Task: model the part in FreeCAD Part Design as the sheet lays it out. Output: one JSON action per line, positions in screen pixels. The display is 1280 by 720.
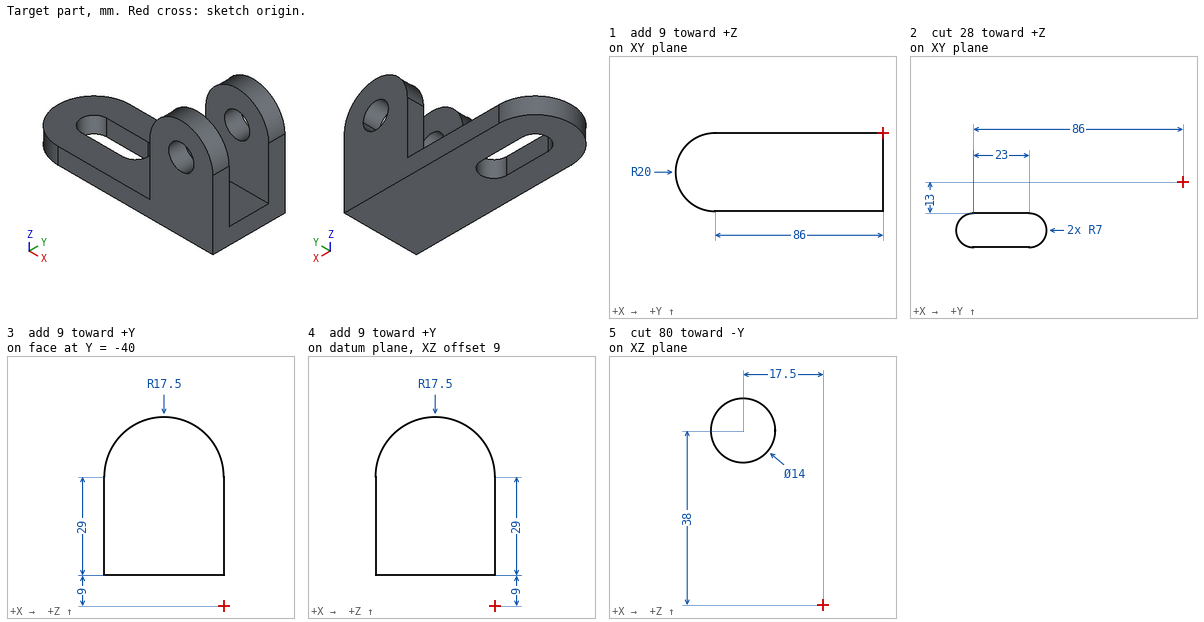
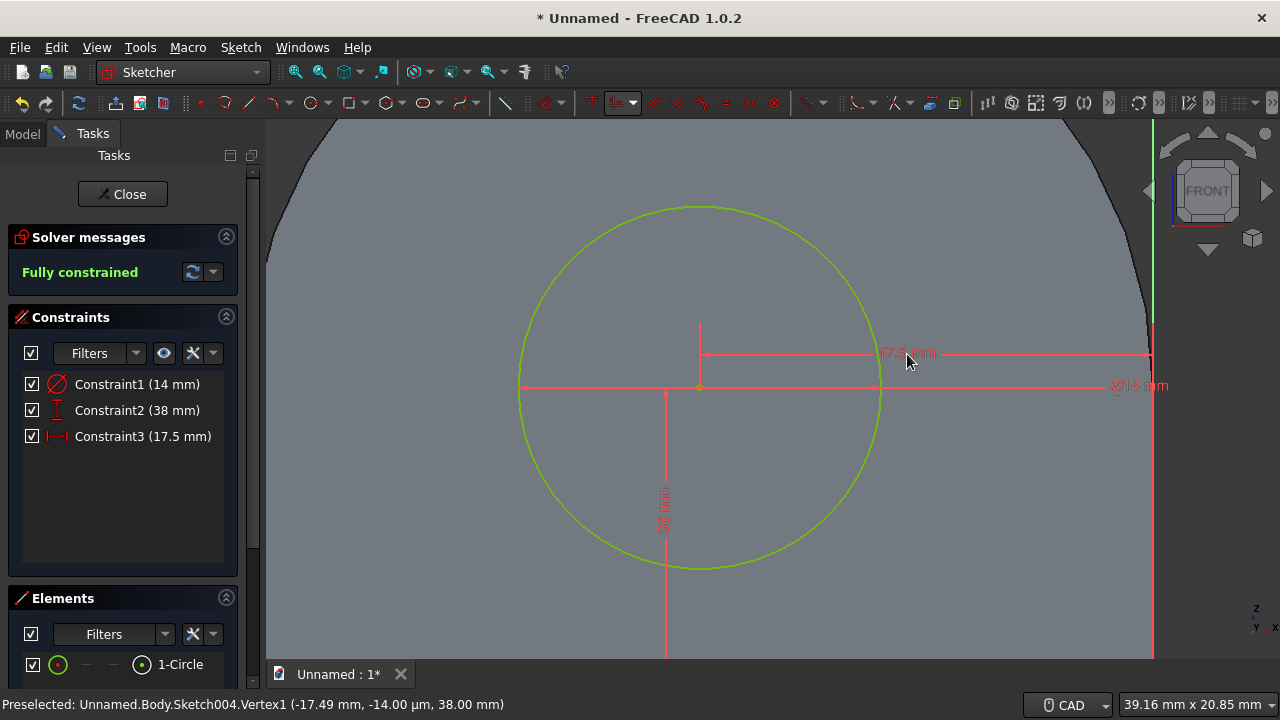
{"action": "left_click", "coordinate": [123, 194]}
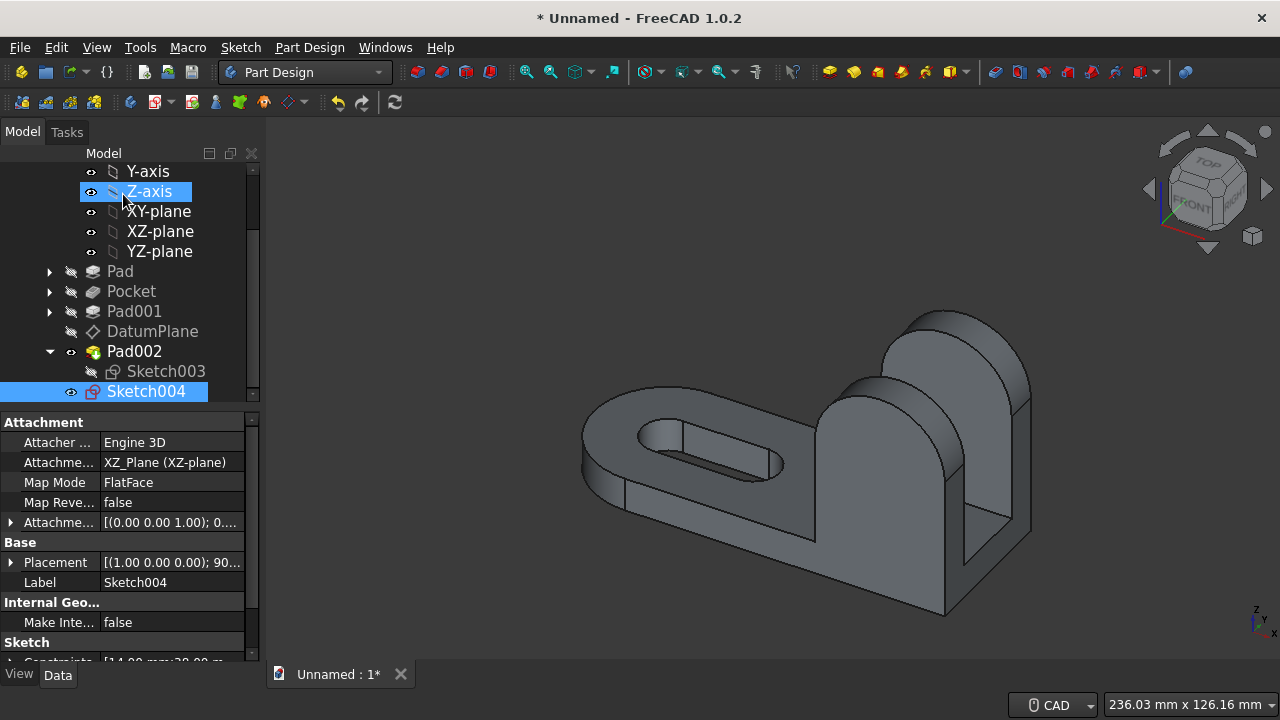
{"action": "left_click", "coordinate": [996, 72]}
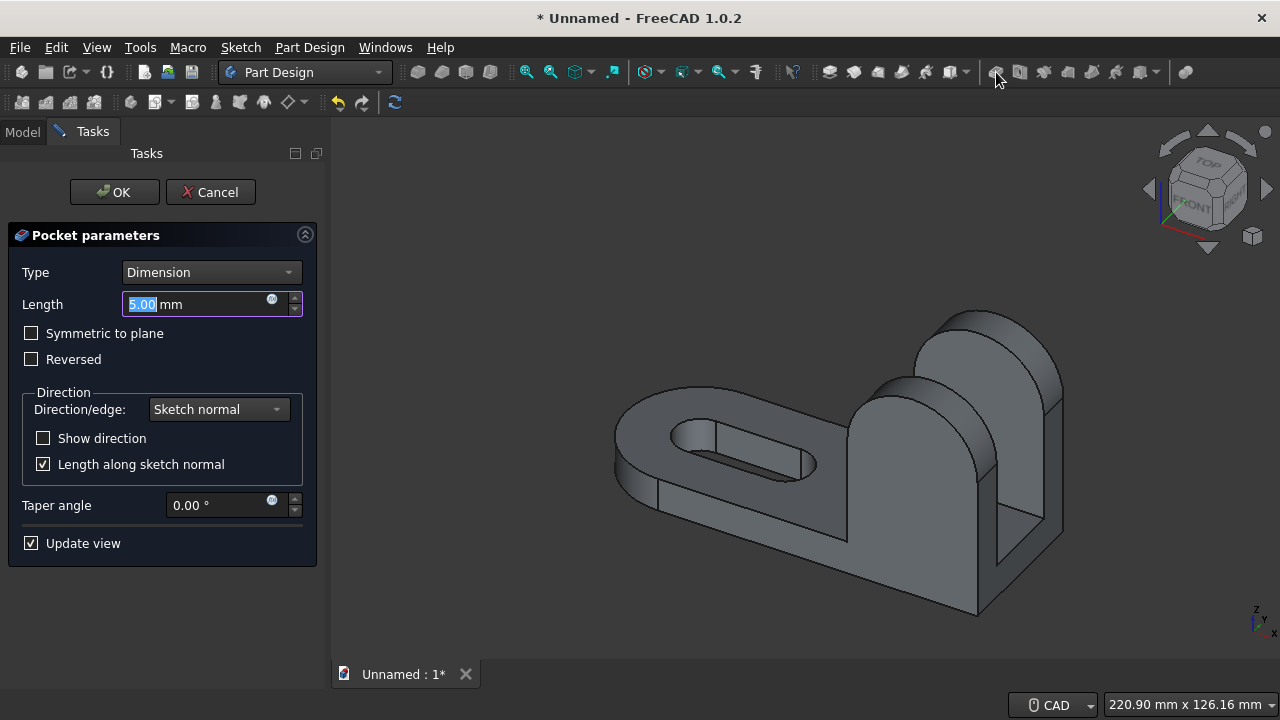
{"action": "type", "text": "80"}
{"action": "key", "text": "Tab"}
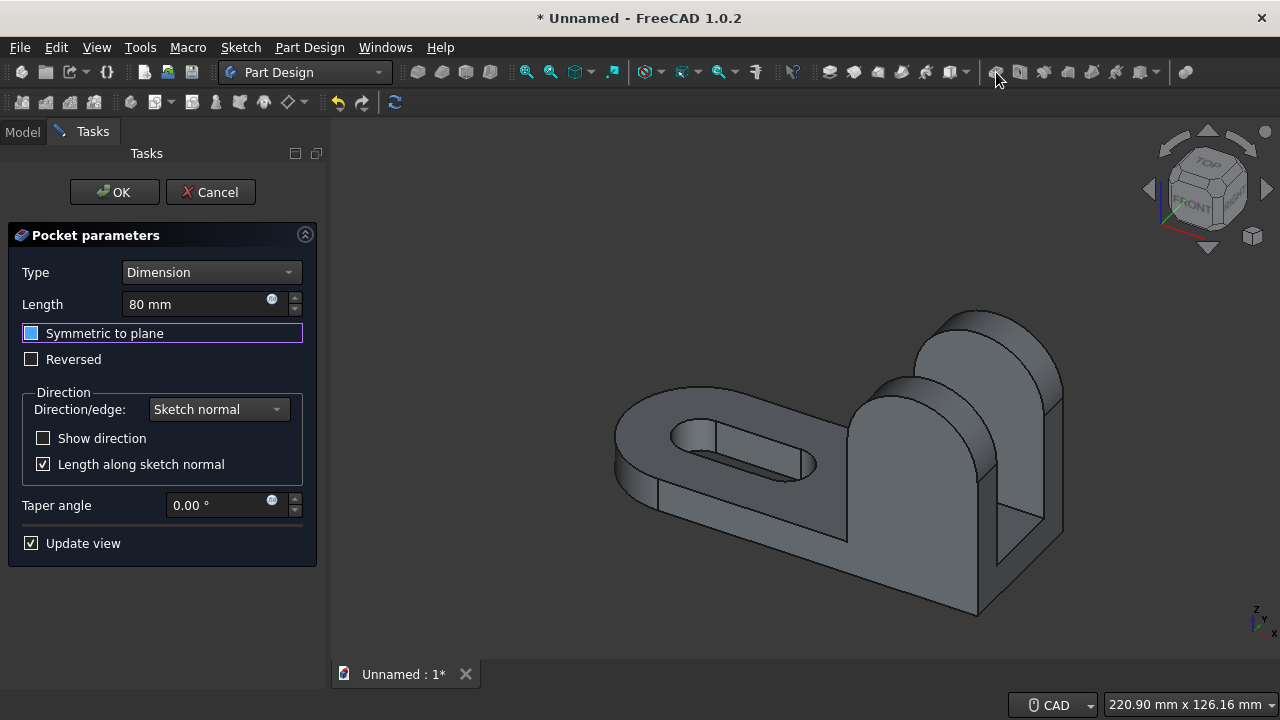
{"action": "left_click", "coordinate": [30, 359]}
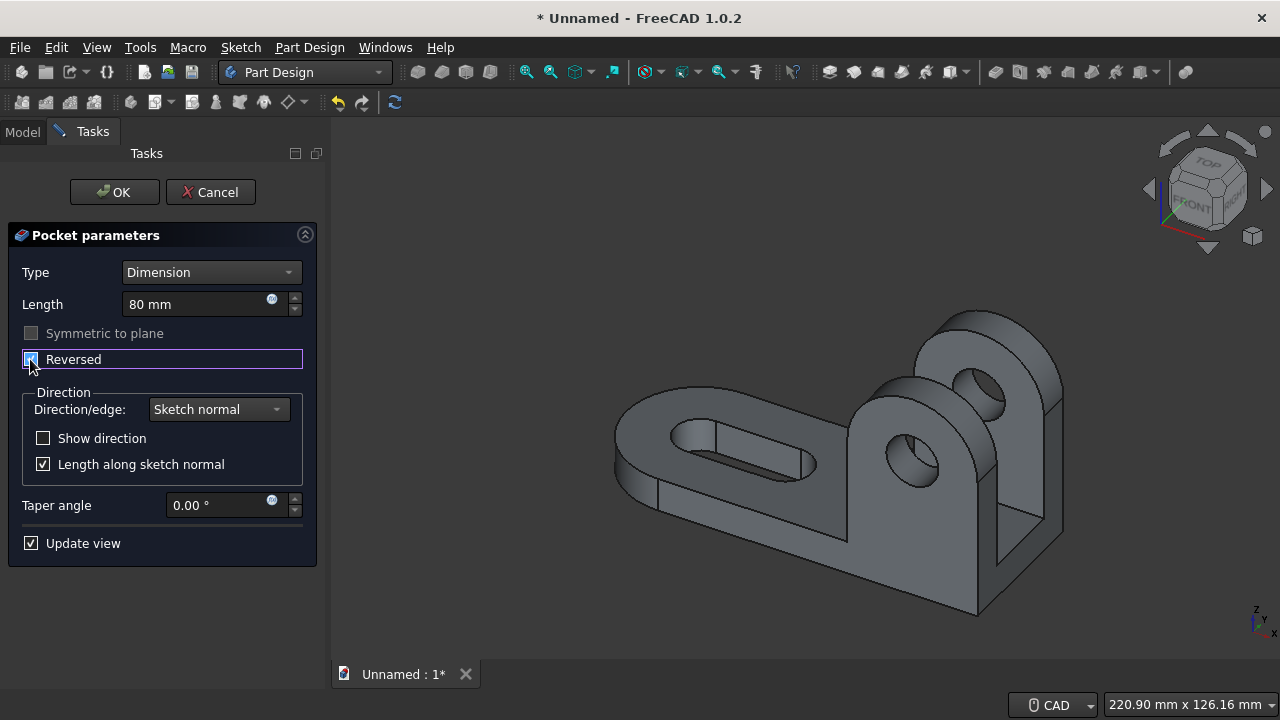
{"action": "left_click", "coordinate": [115, 192]}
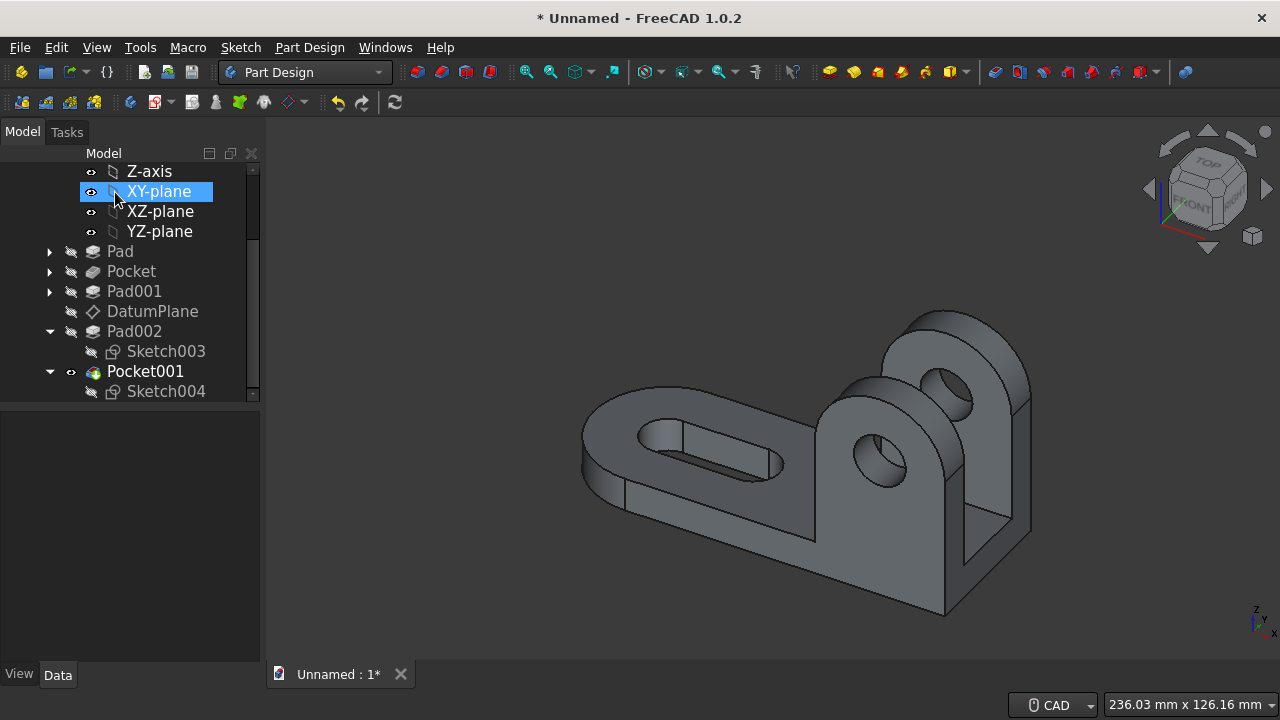
{"action": "key", "text": "0"}